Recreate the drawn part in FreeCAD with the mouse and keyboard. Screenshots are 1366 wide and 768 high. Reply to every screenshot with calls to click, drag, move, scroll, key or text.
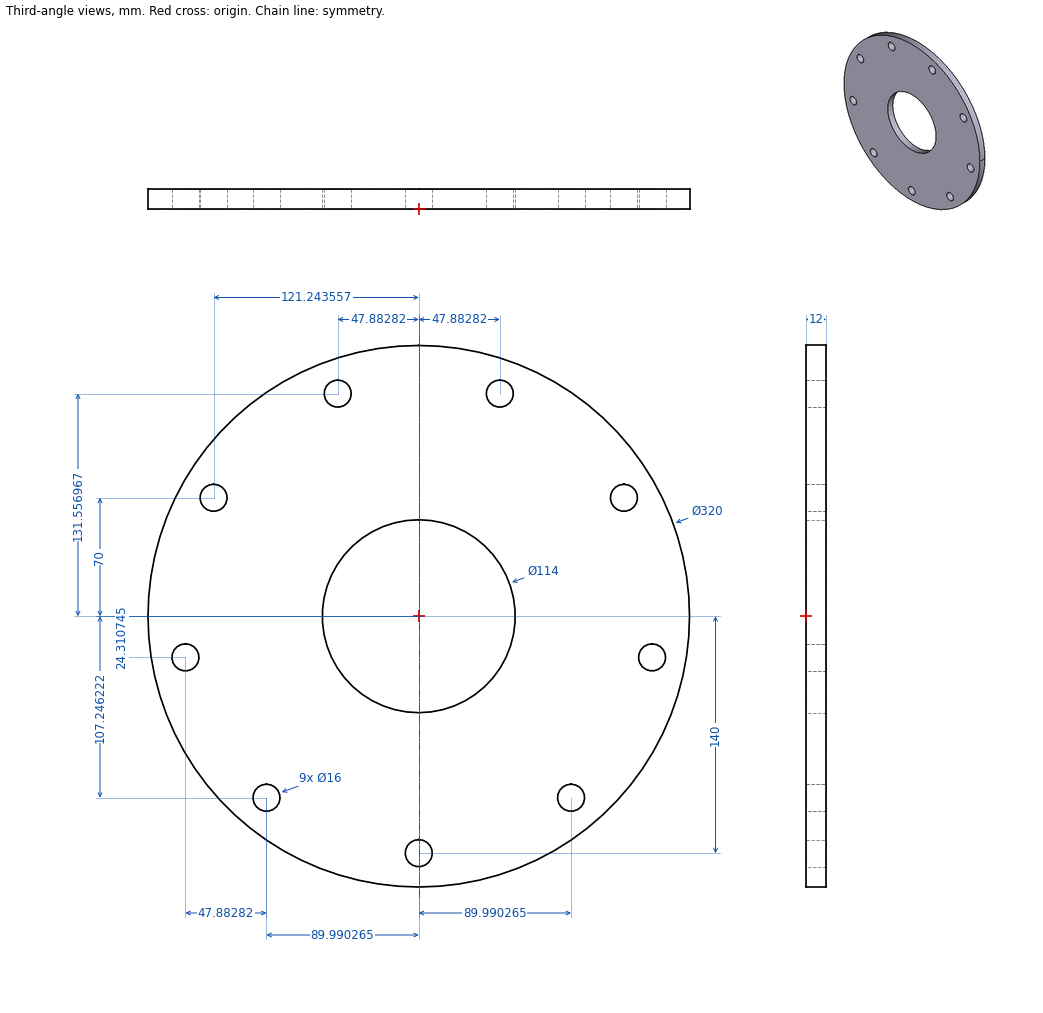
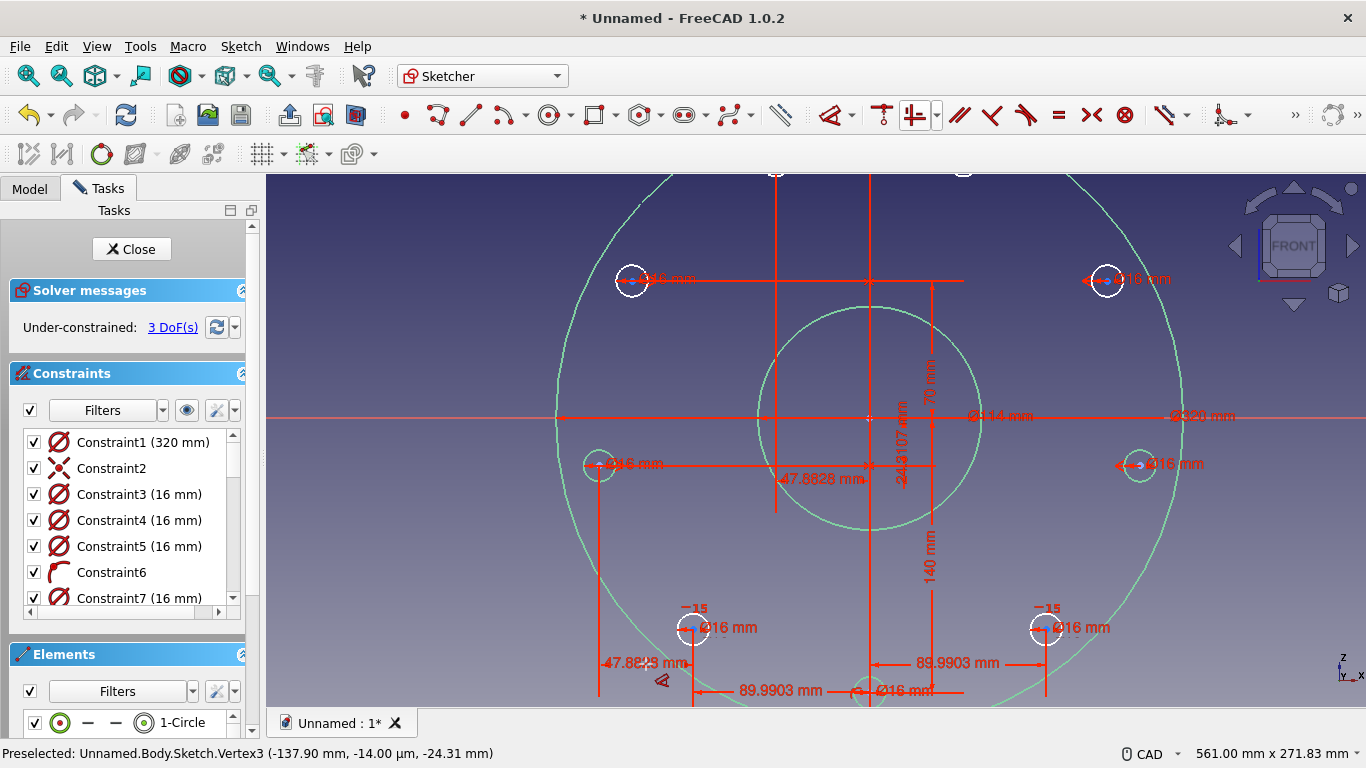
click(693, 630)
click(659, 524)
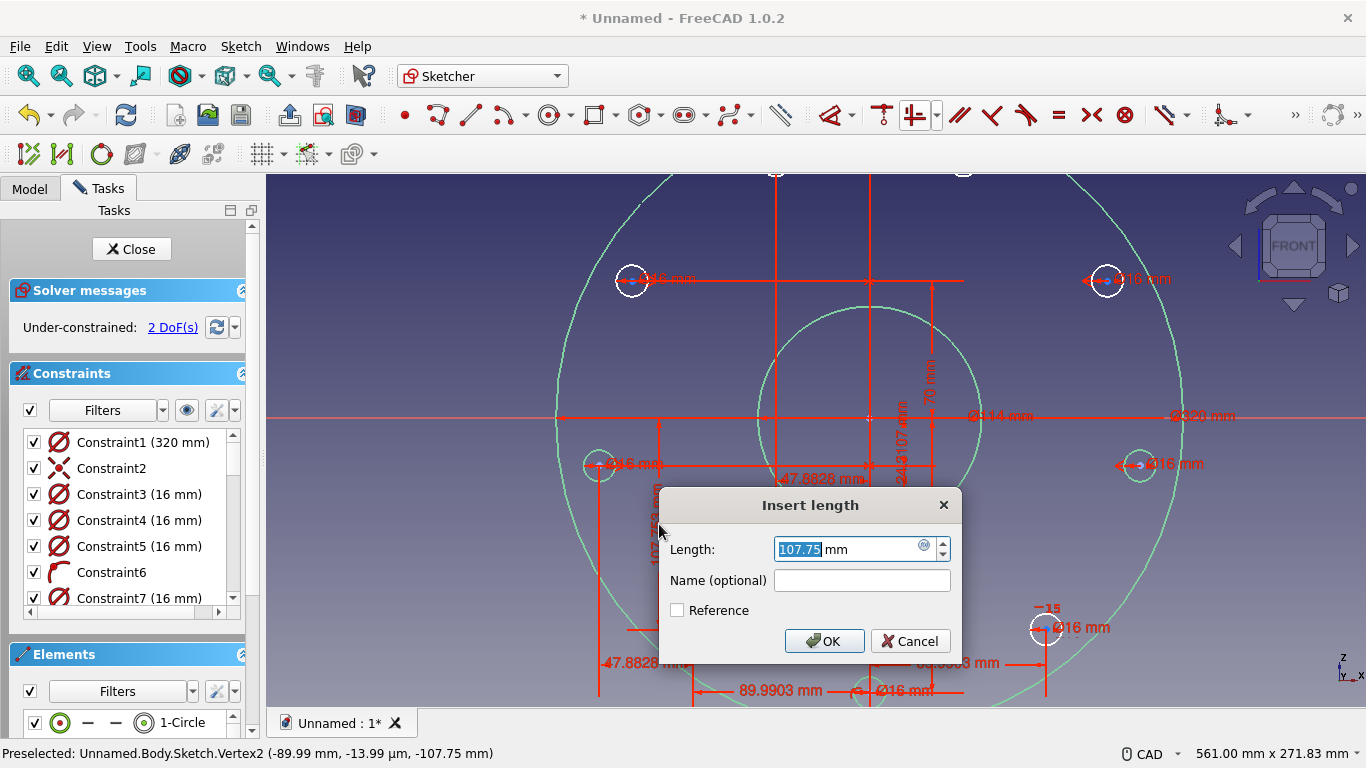
text(107.246222)
key(Return)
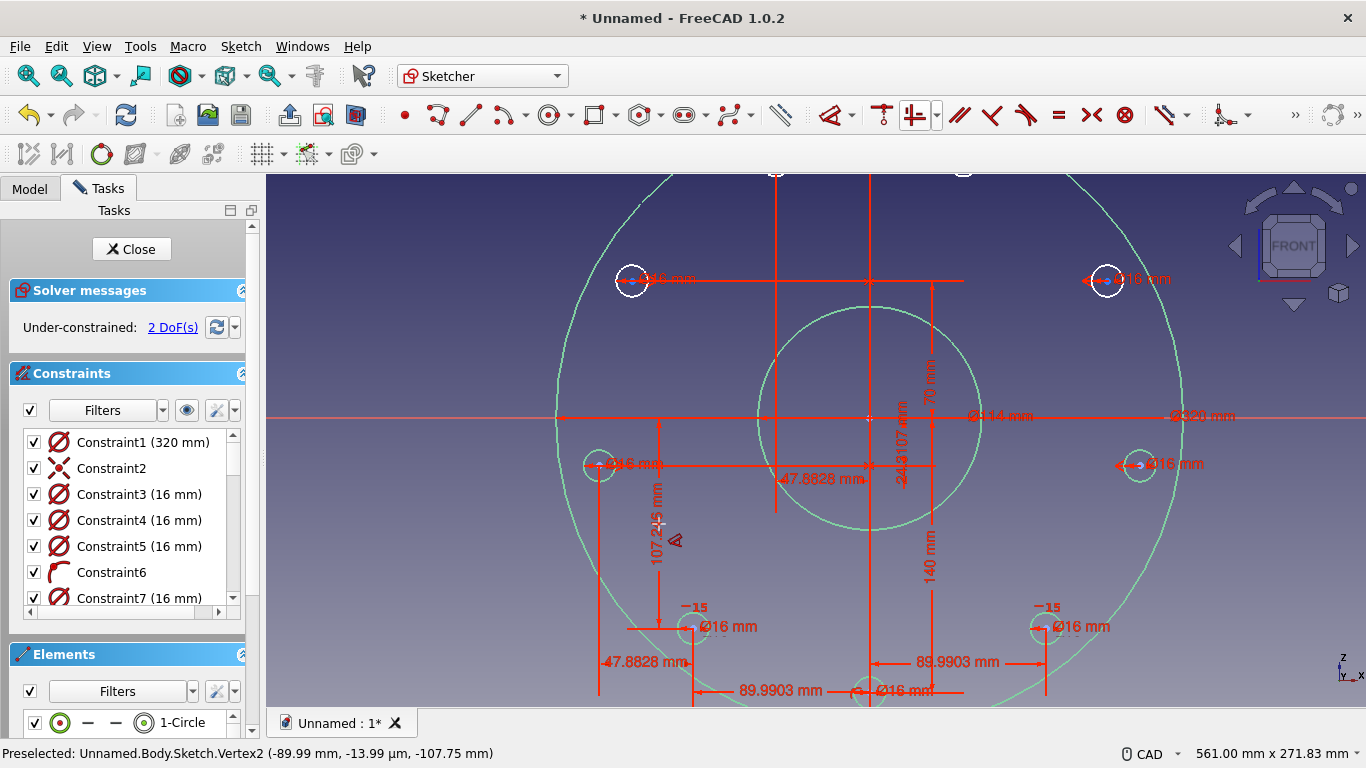
click(632, 281)
click(751, 247)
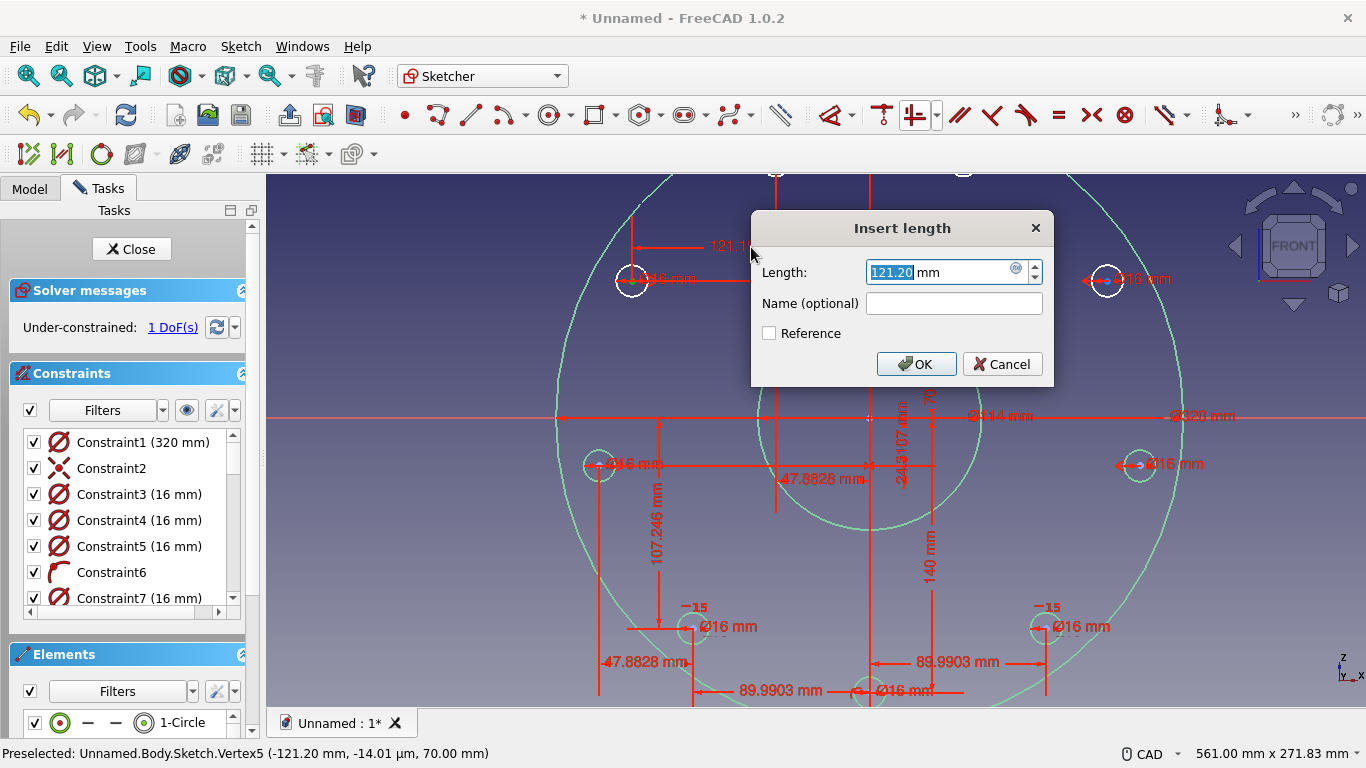
text(121.243557)
key(Return)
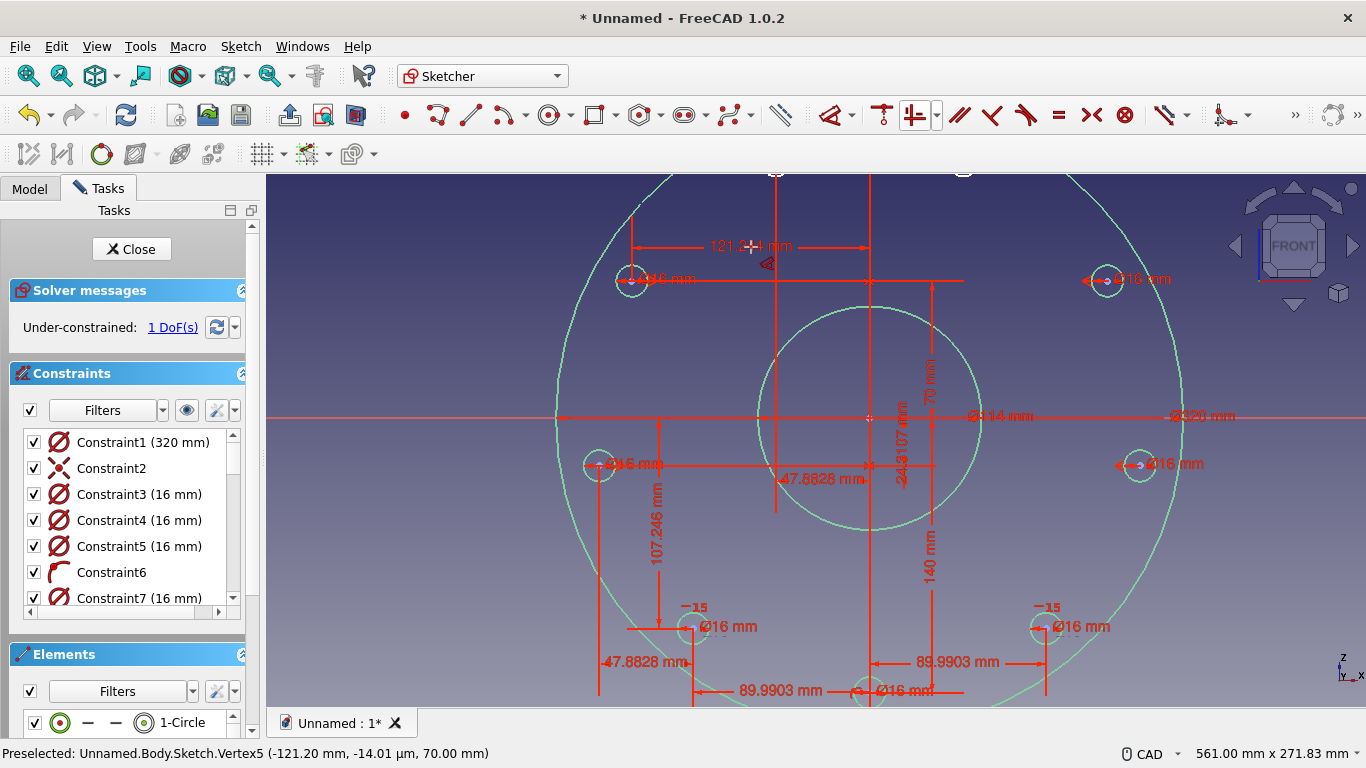
scroll(599, 468, down, 3)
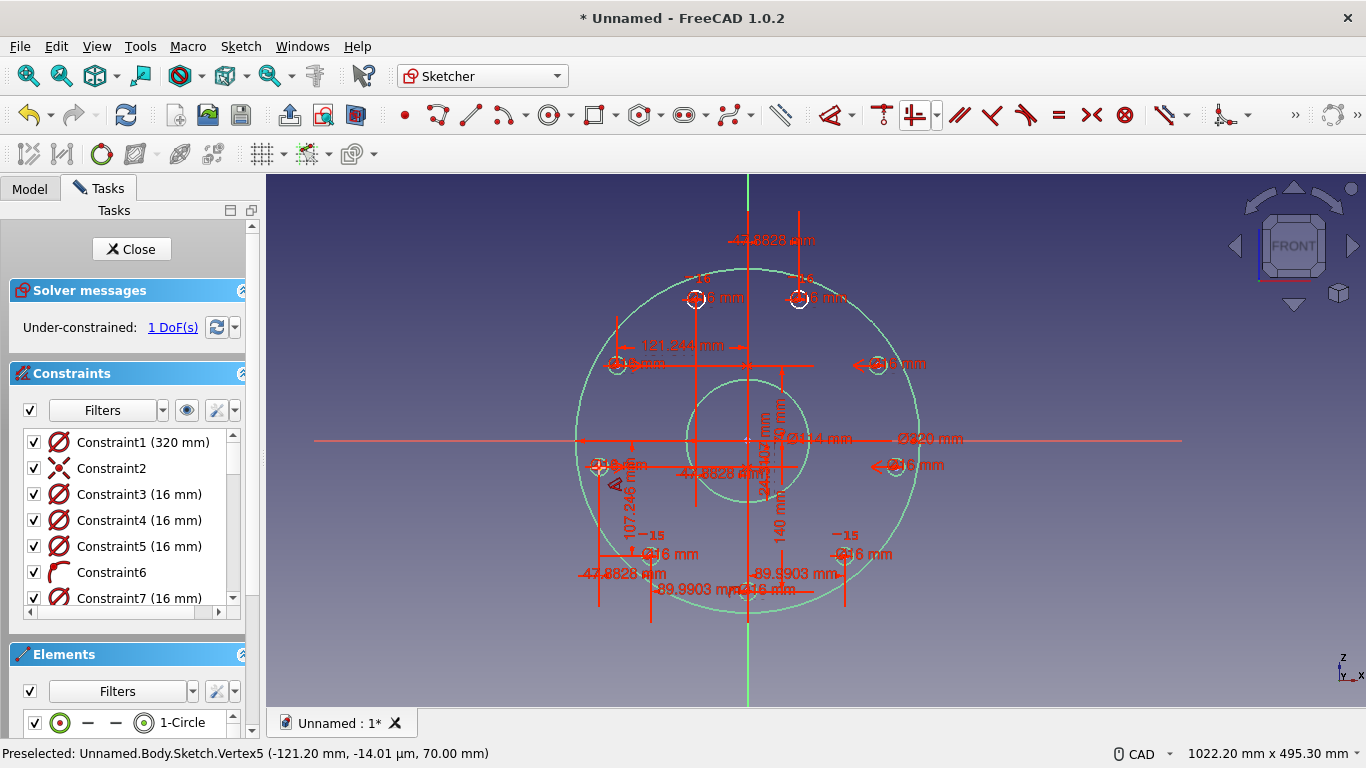
click(696, 300)
click(662, 370)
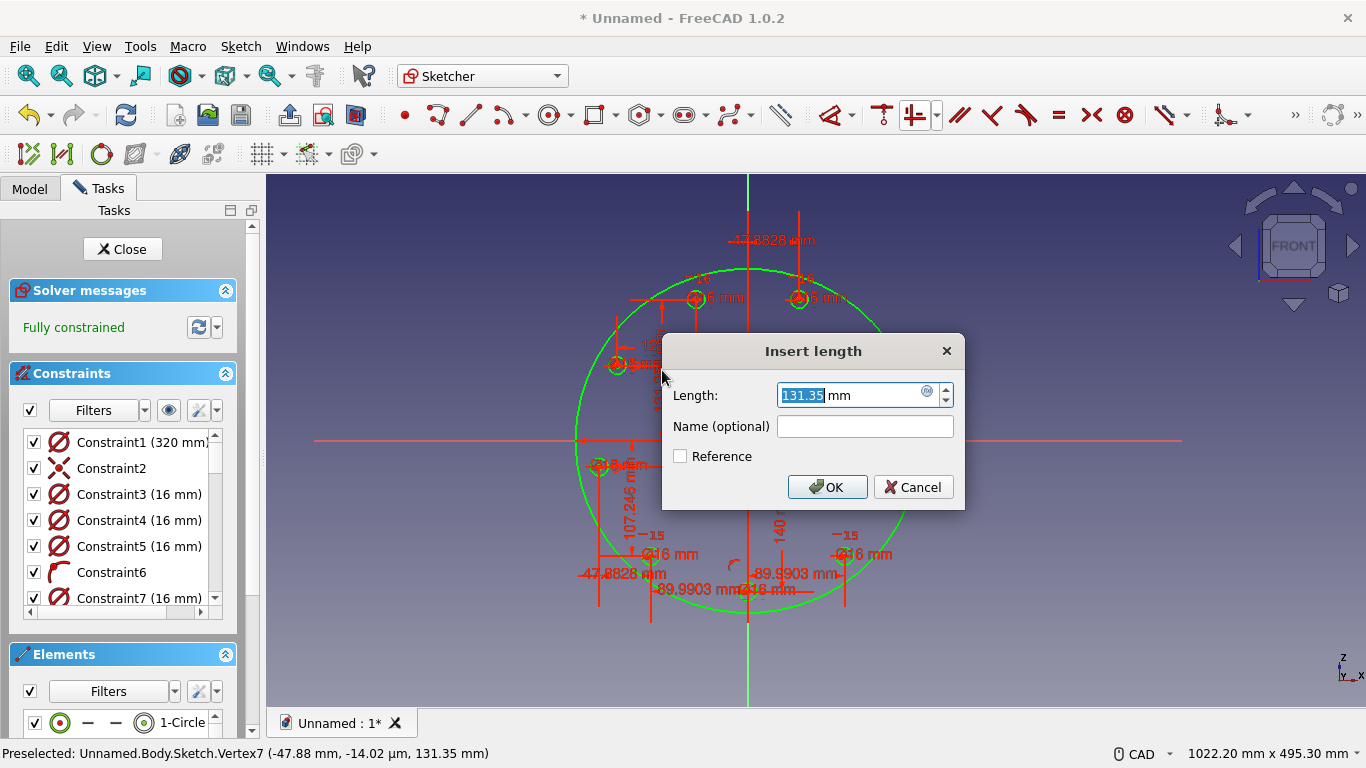
text(131.556967)
key(Return)
key(Escape)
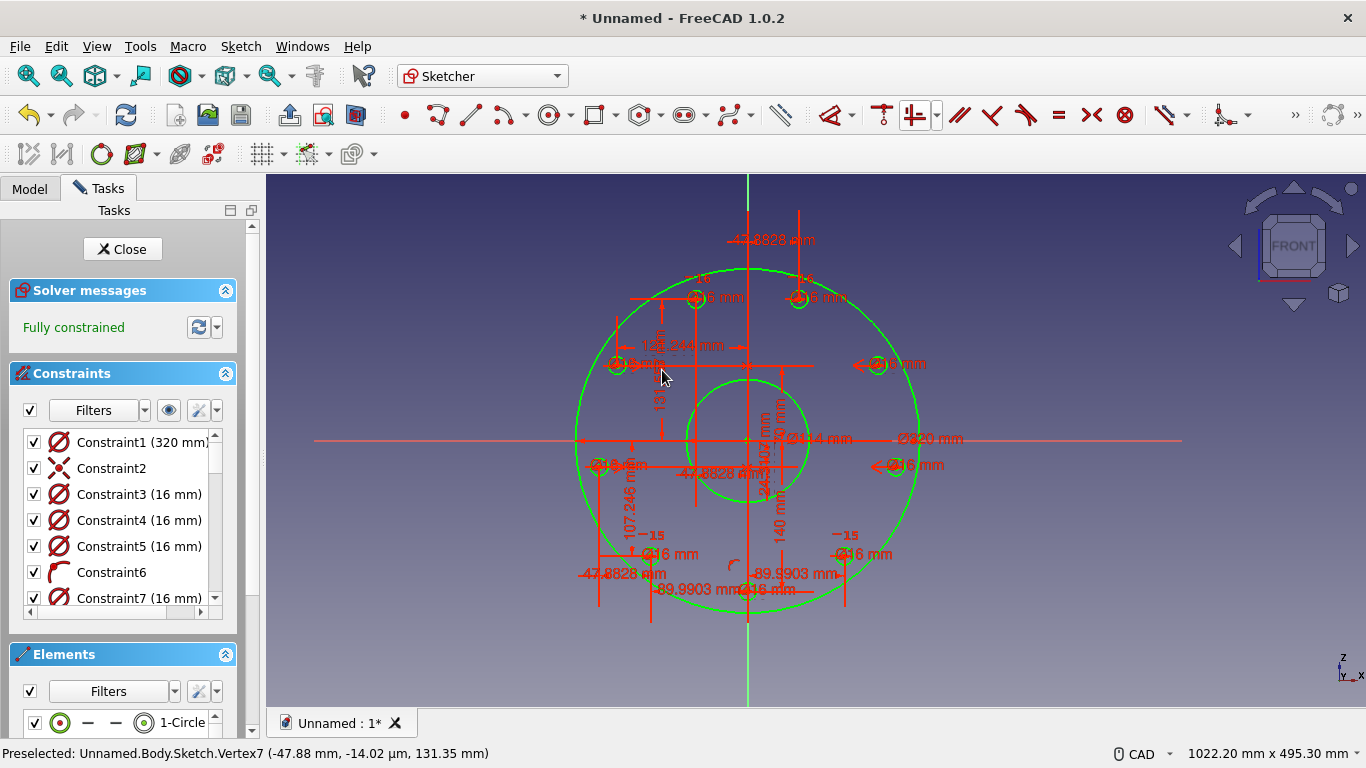
click(123, 249)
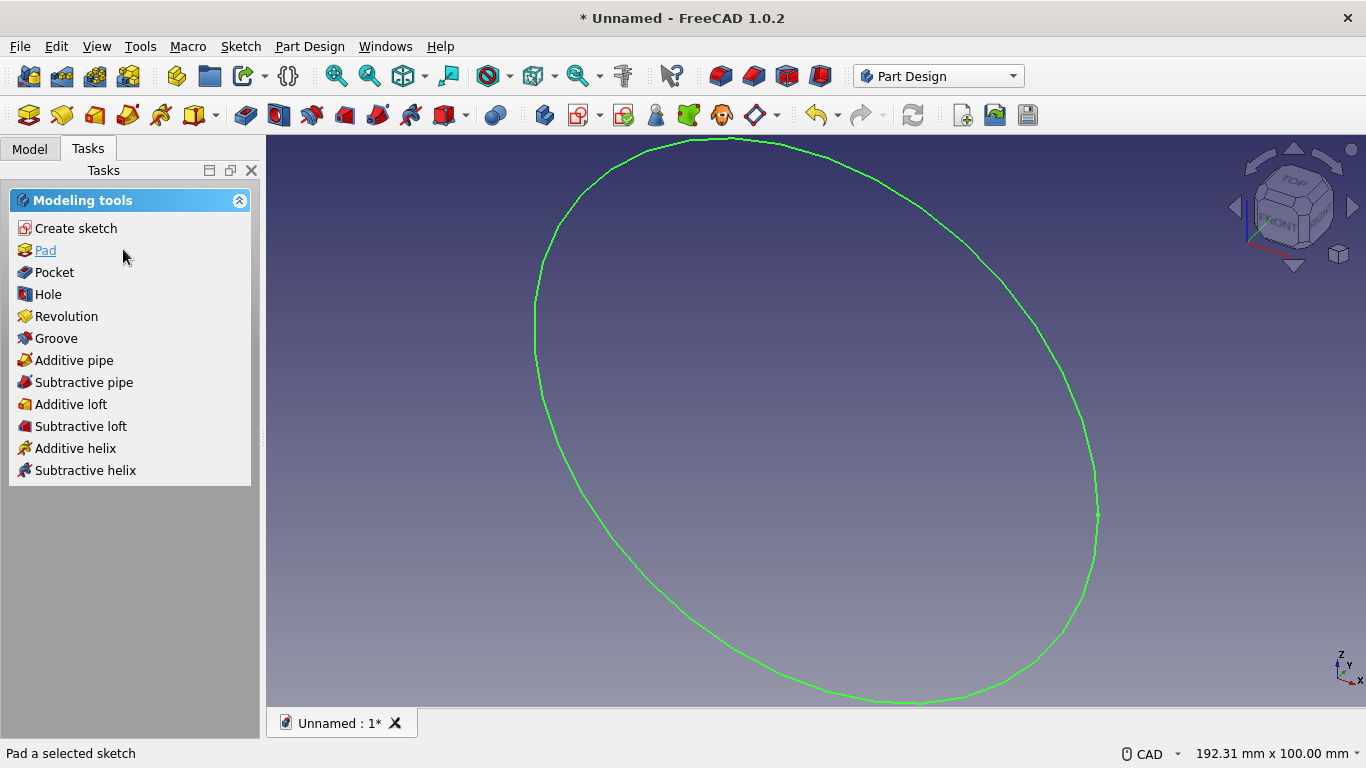
click(29, 116)